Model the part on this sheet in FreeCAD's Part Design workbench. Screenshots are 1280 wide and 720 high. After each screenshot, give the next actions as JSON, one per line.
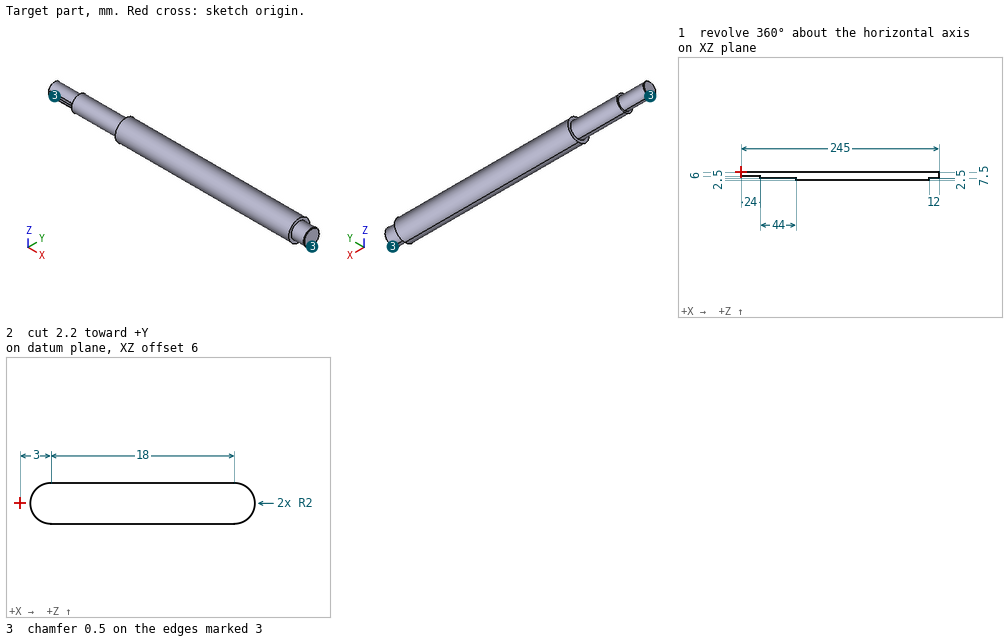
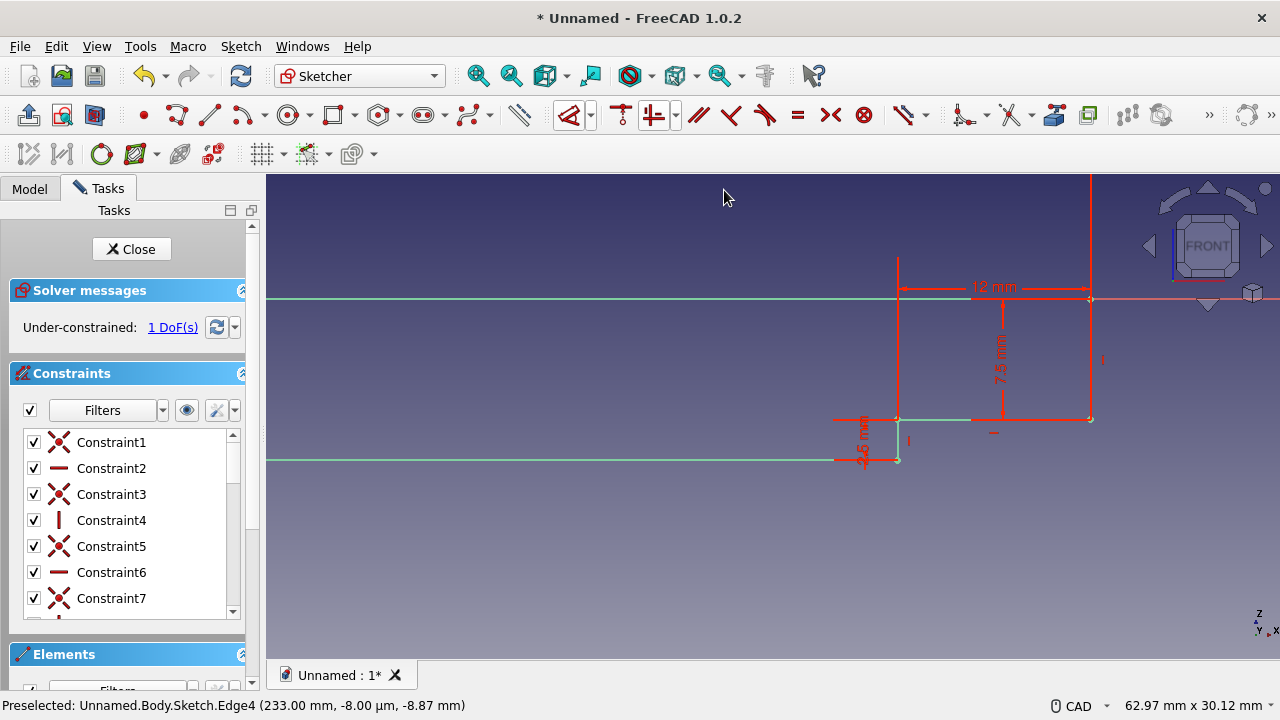
{"action": "scroll", "coordinate": [953, 422], "scroll_direction": "down", "scroll_amount": 10}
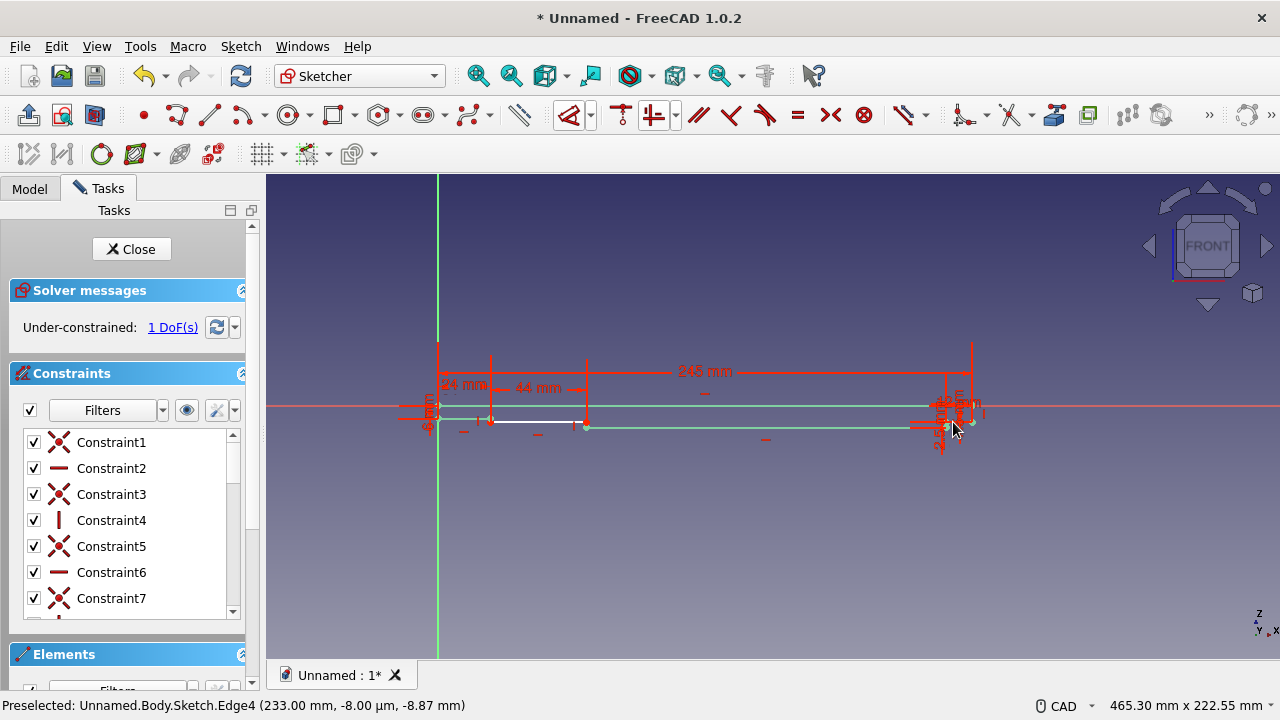
{"action": "scroll", "coordinate": [587, 426], "scroll_direction": "up", "scroll_amount": 11}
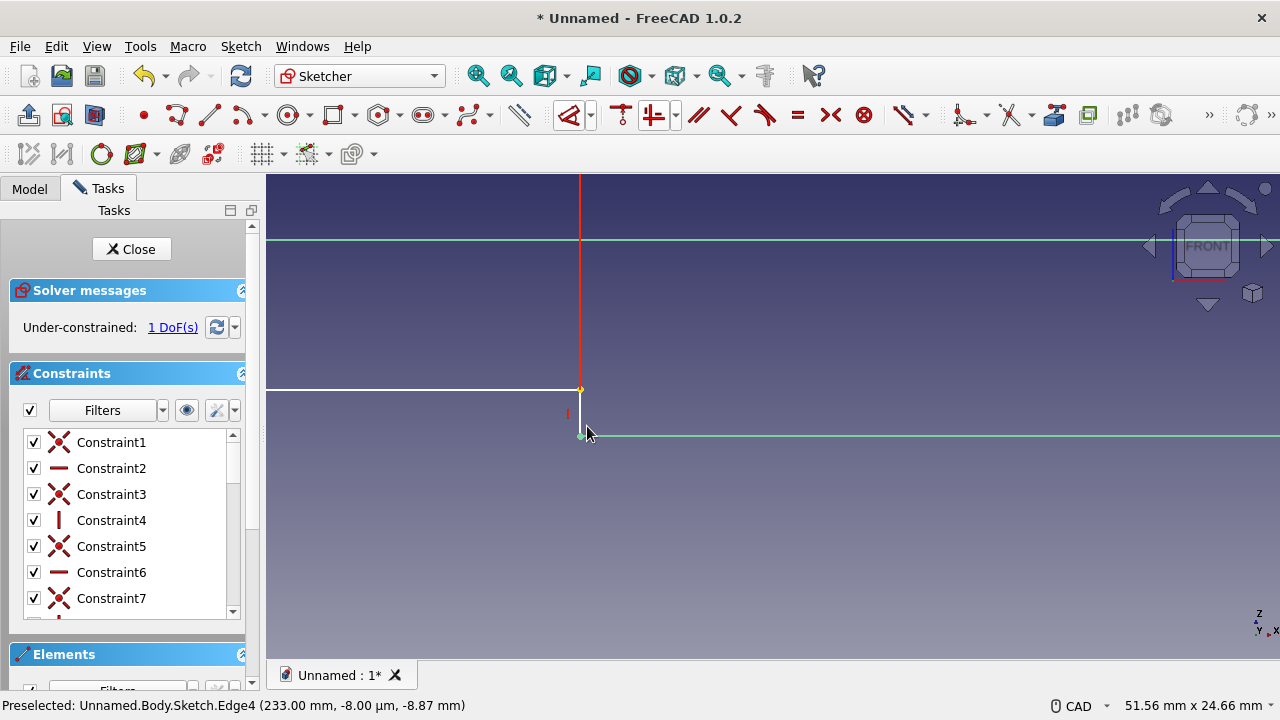
{"action": "left_click", "coordinate": [580, 422]}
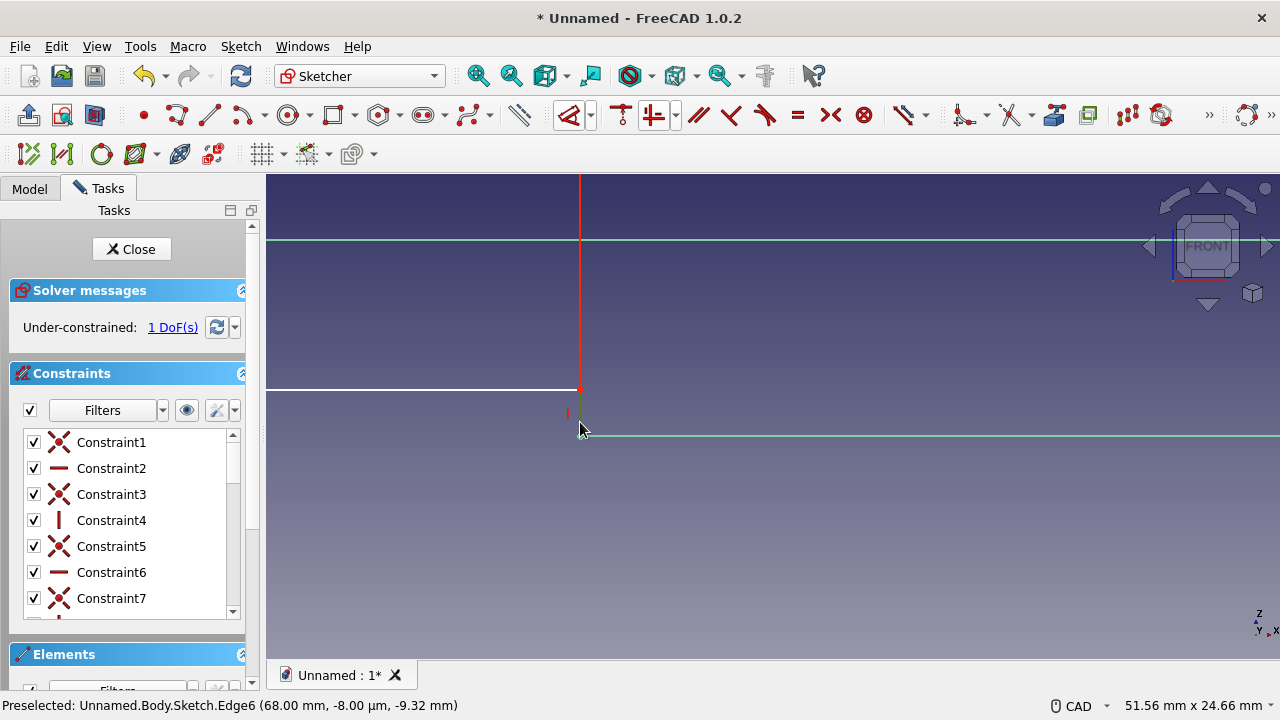
{"action": "left_click", "coordinate": [590, 116]}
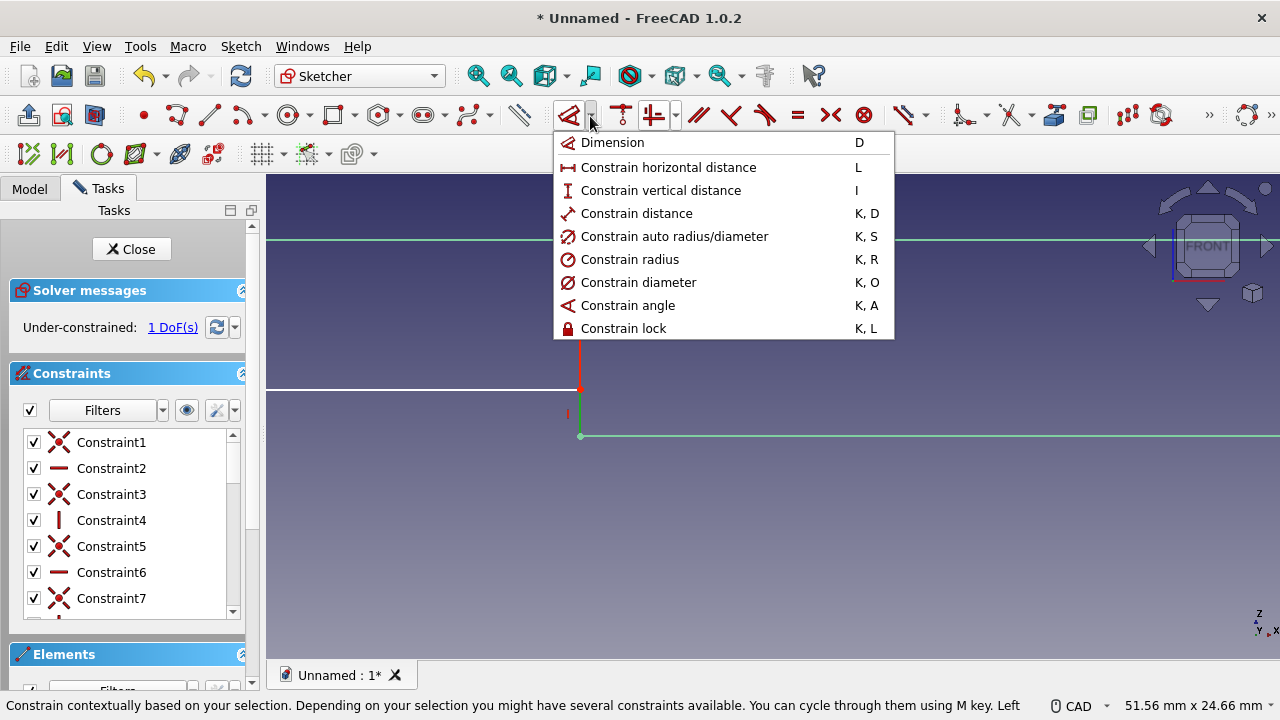
{"action": "left_click", "coordinate": [724, 190]}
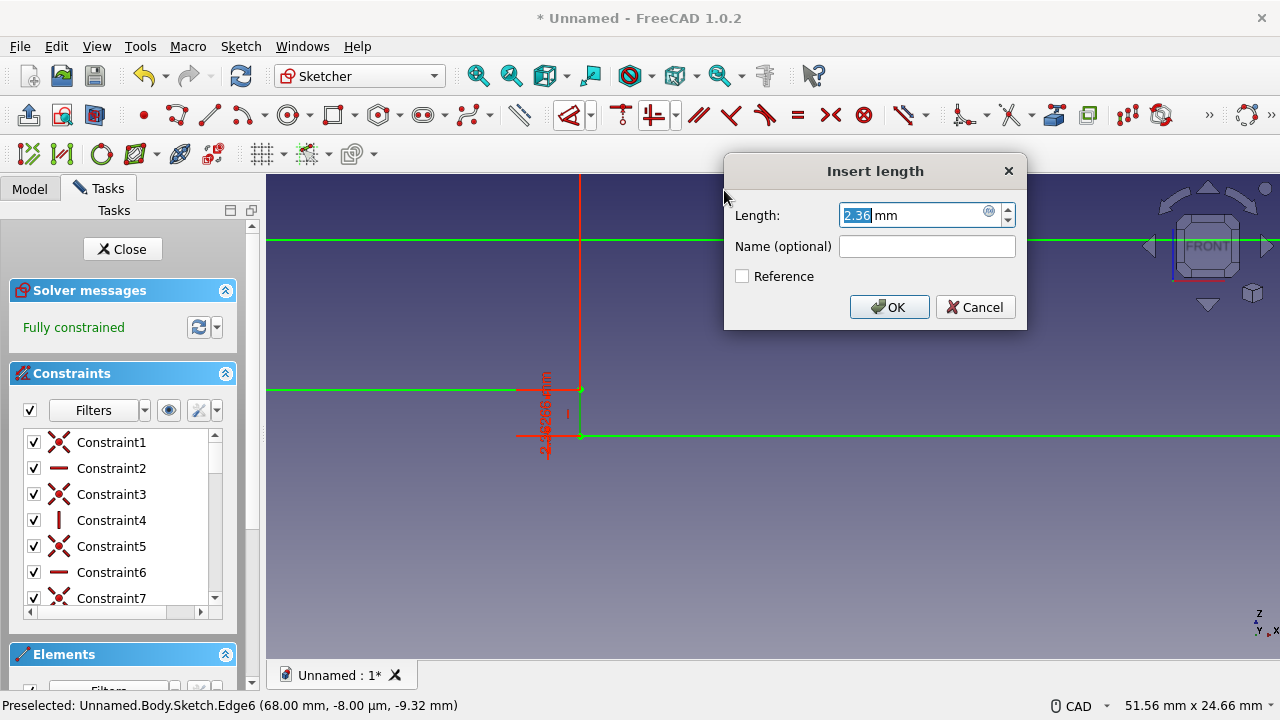
{"action": "type", "text": "2.5"}
{"action": "key", "text": "Return"}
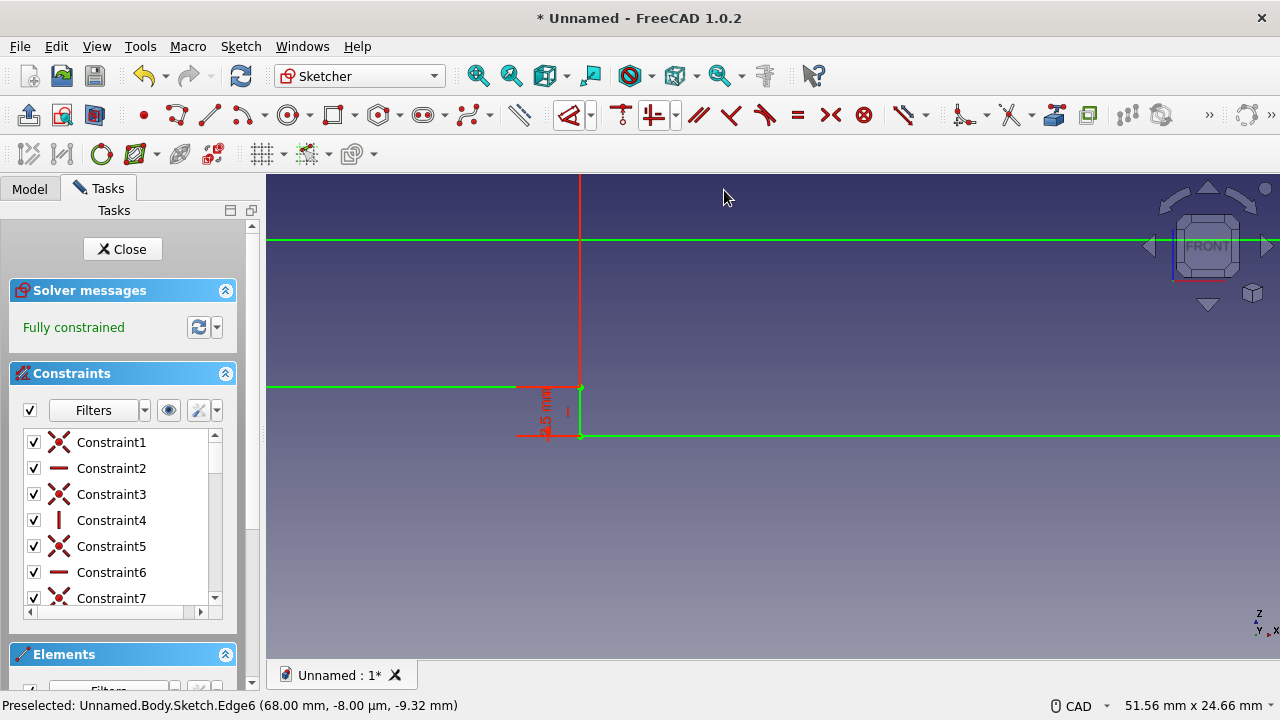
{"action": "left_click", "coordinate": [123, 249]}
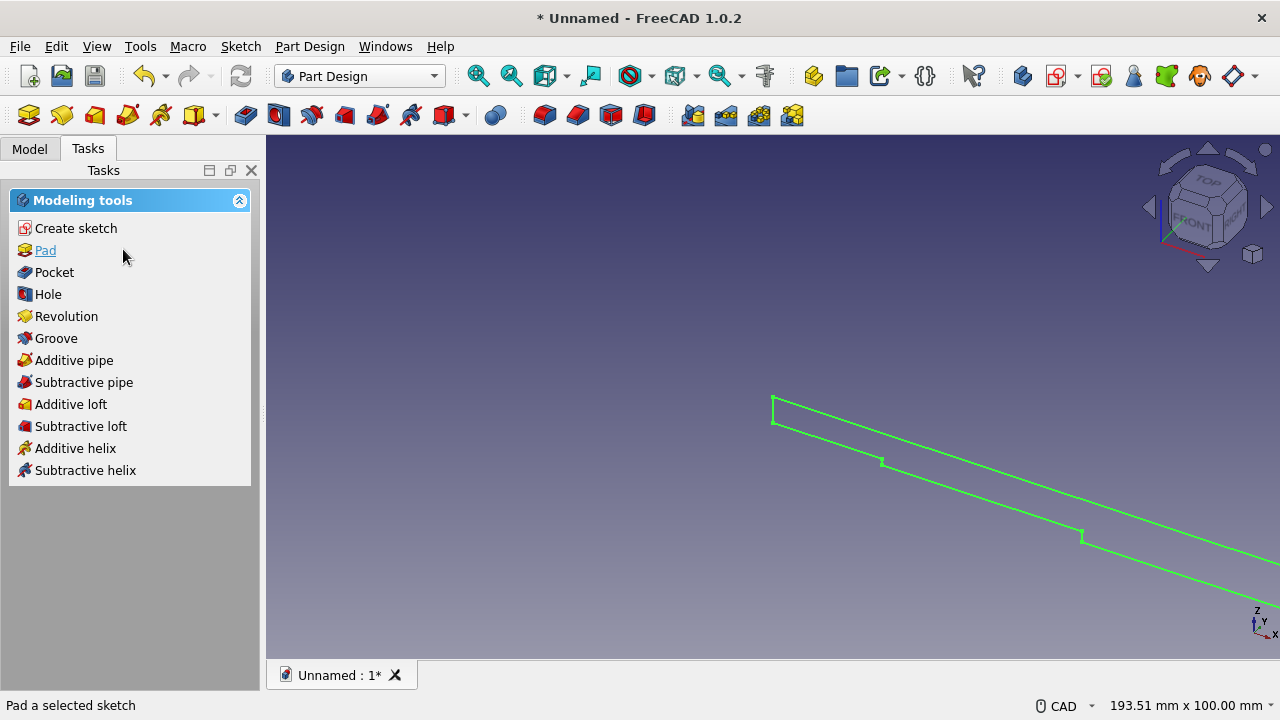
{"action": "left_click", "coordinate": [62, 116]}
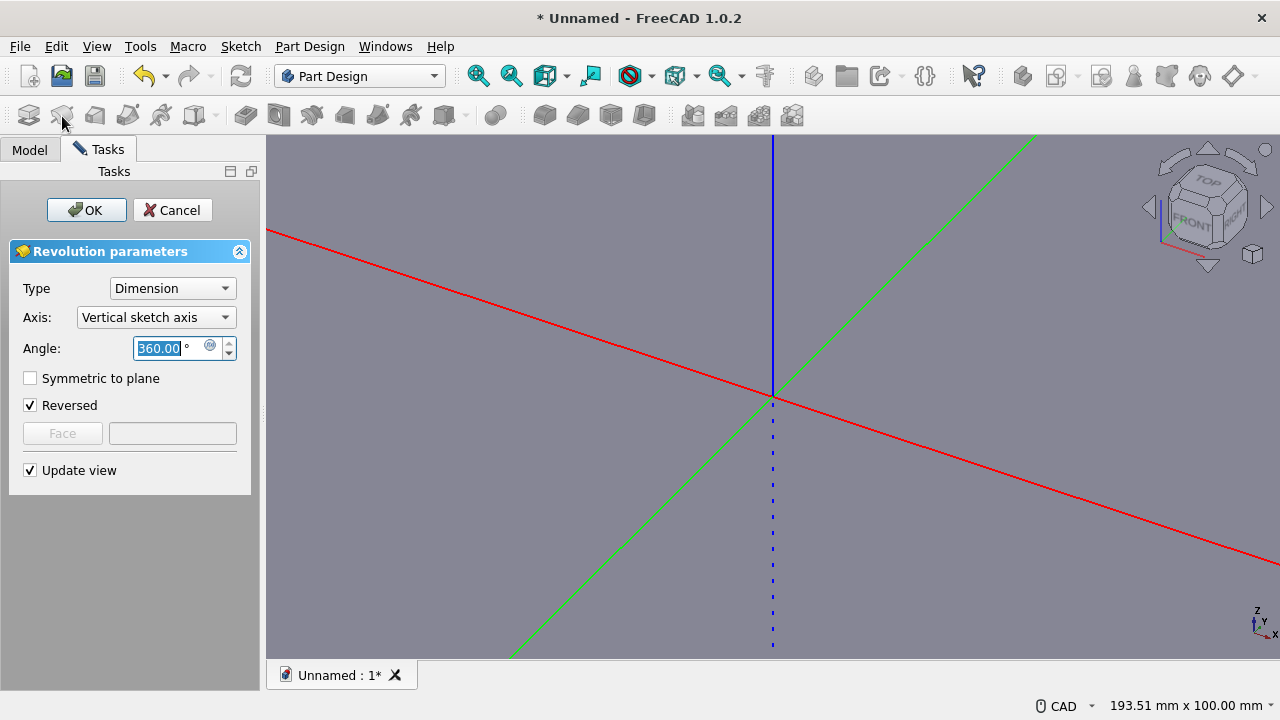
{"action": "left_click", "coordinate": [157, 318]}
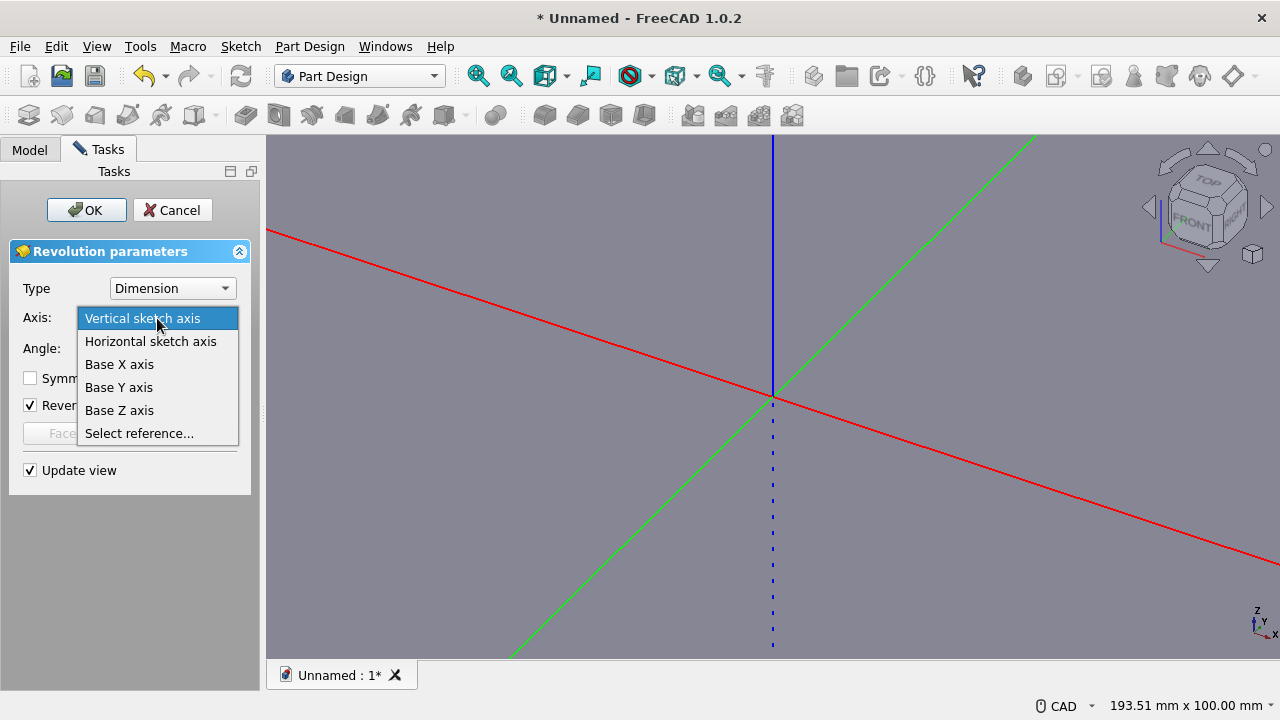
{"action": "left_click", "coordinate": [156, 342]}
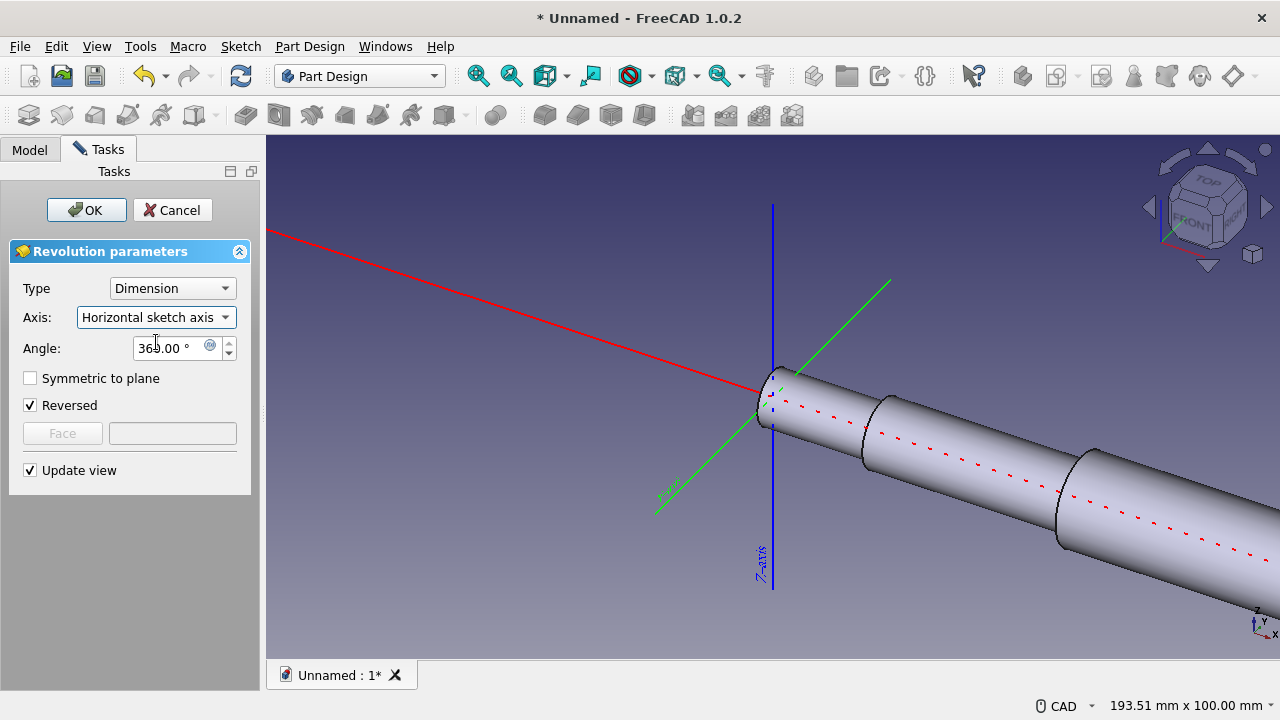
{"action": "left_click", "coordinate": [87, 210]}